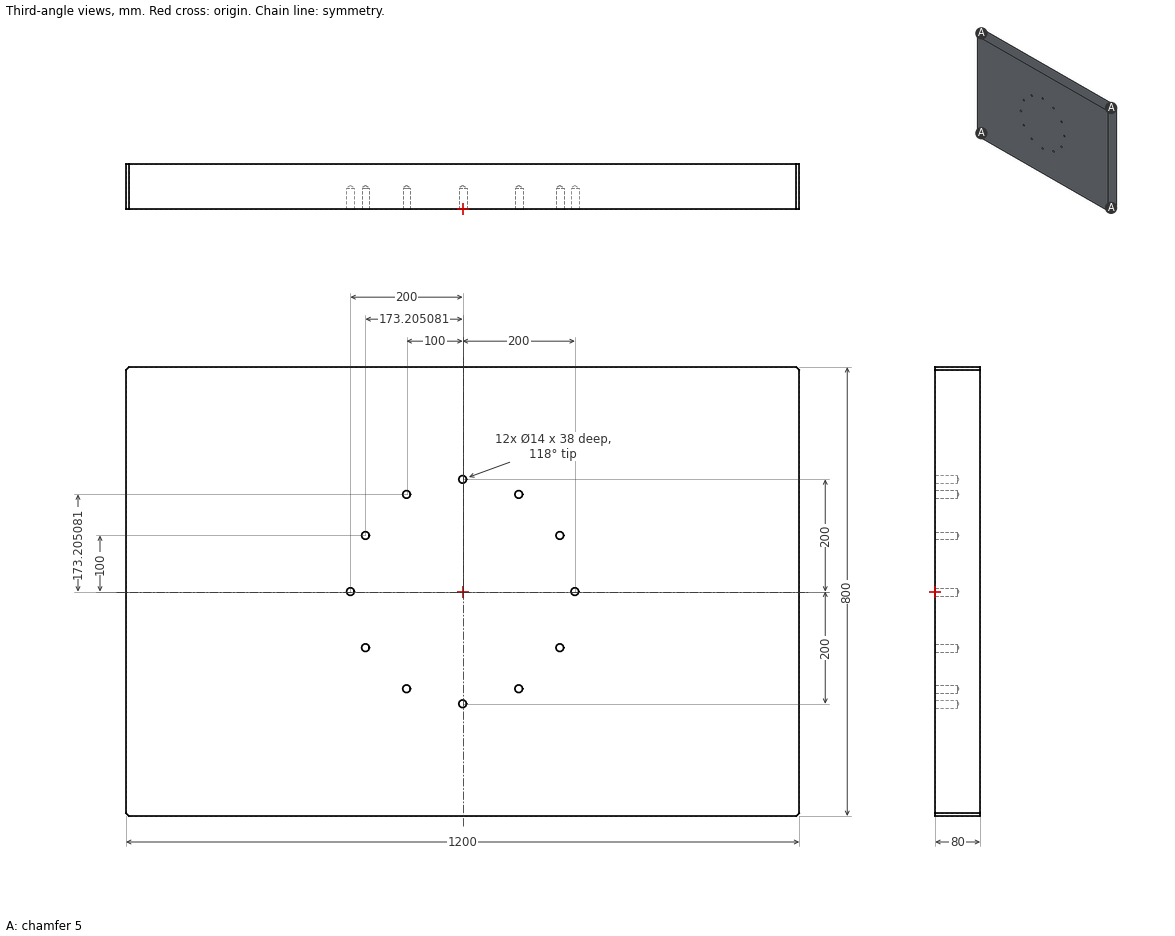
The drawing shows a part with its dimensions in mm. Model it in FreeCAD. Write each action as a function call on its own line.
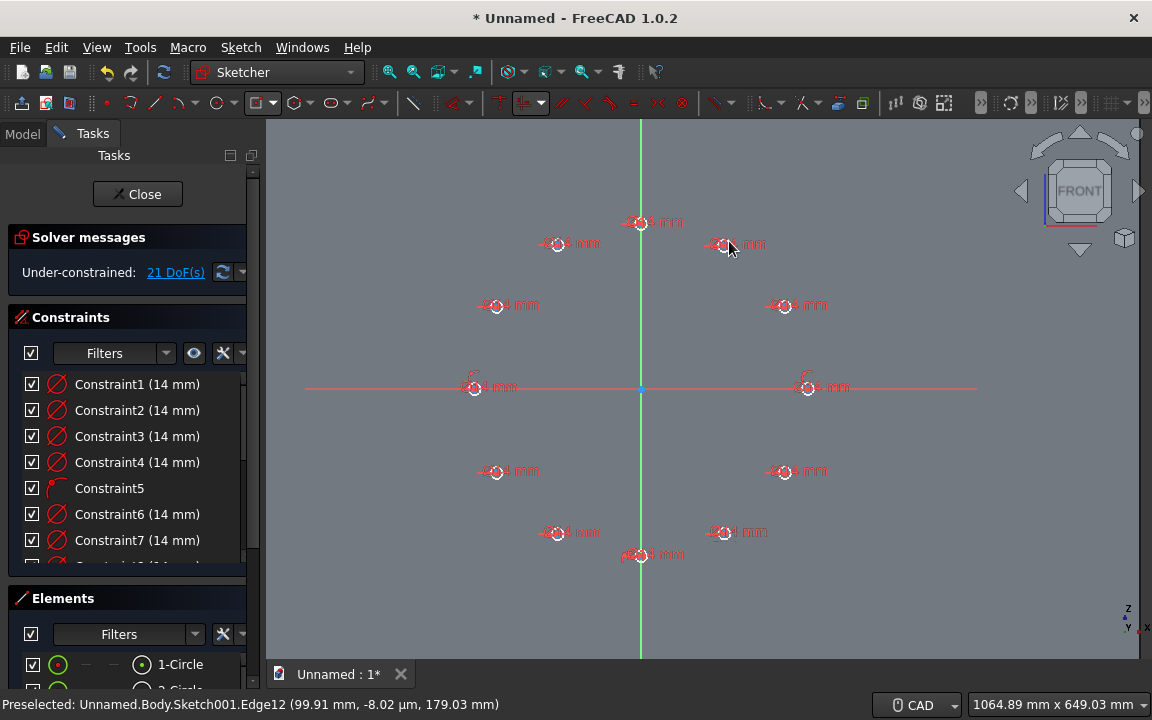
click(641, 224)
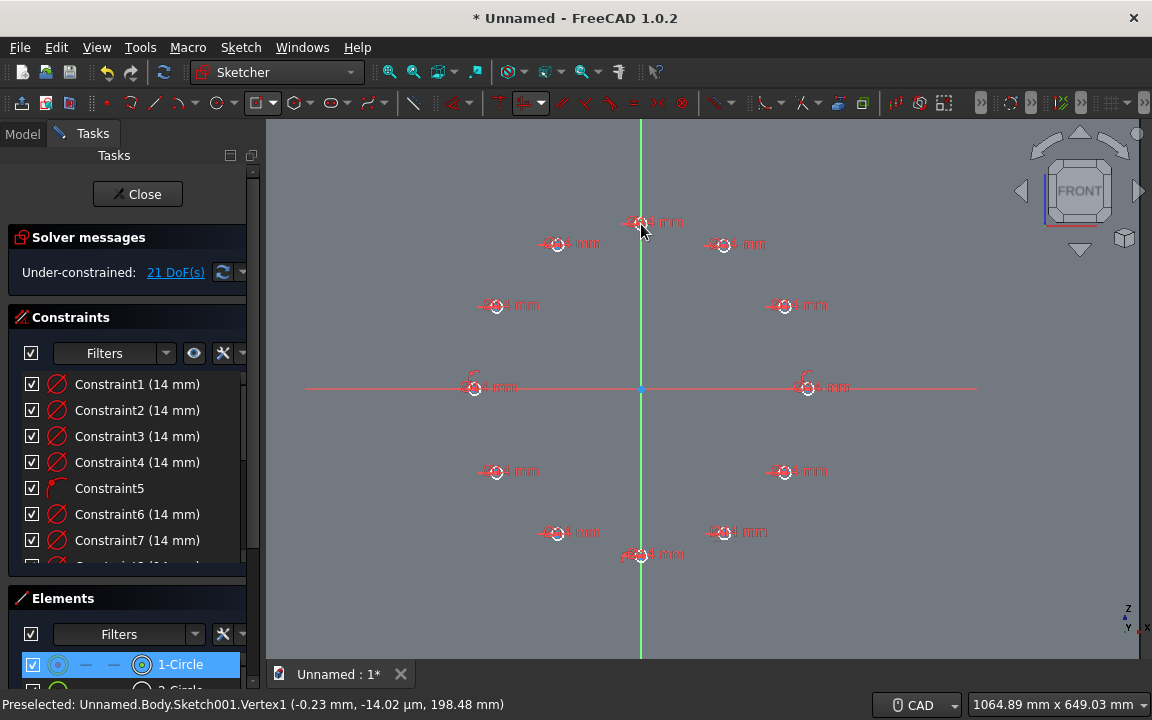
click(641, 596)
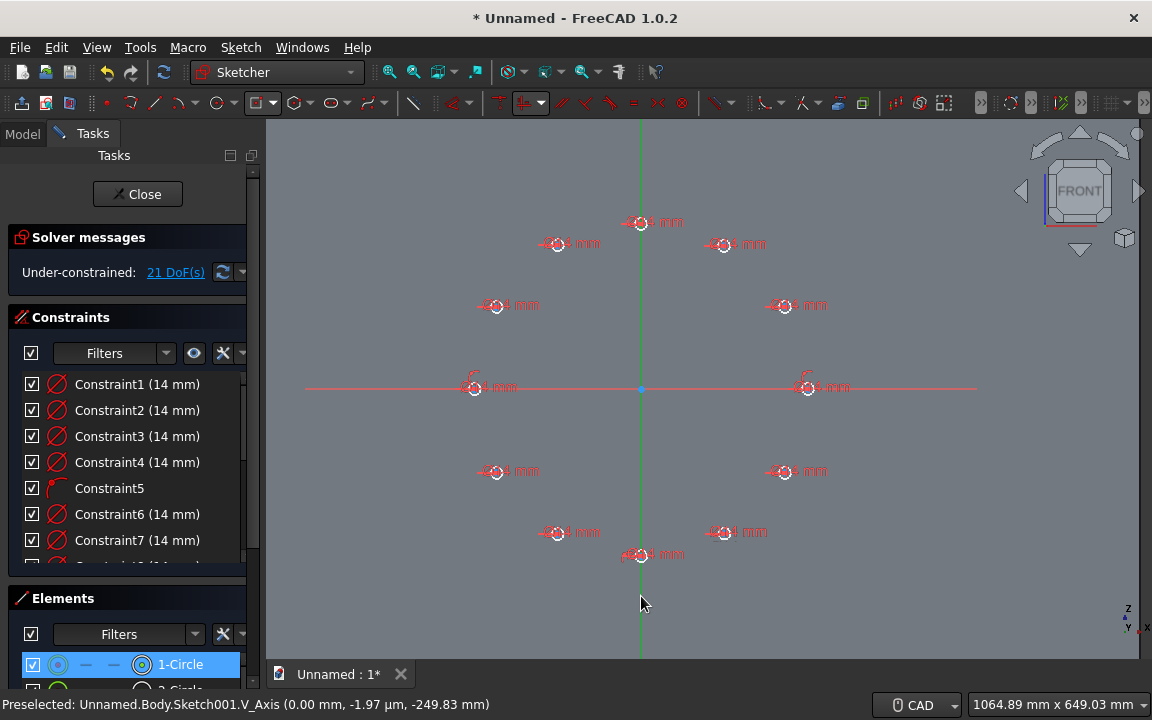
click(500, 104)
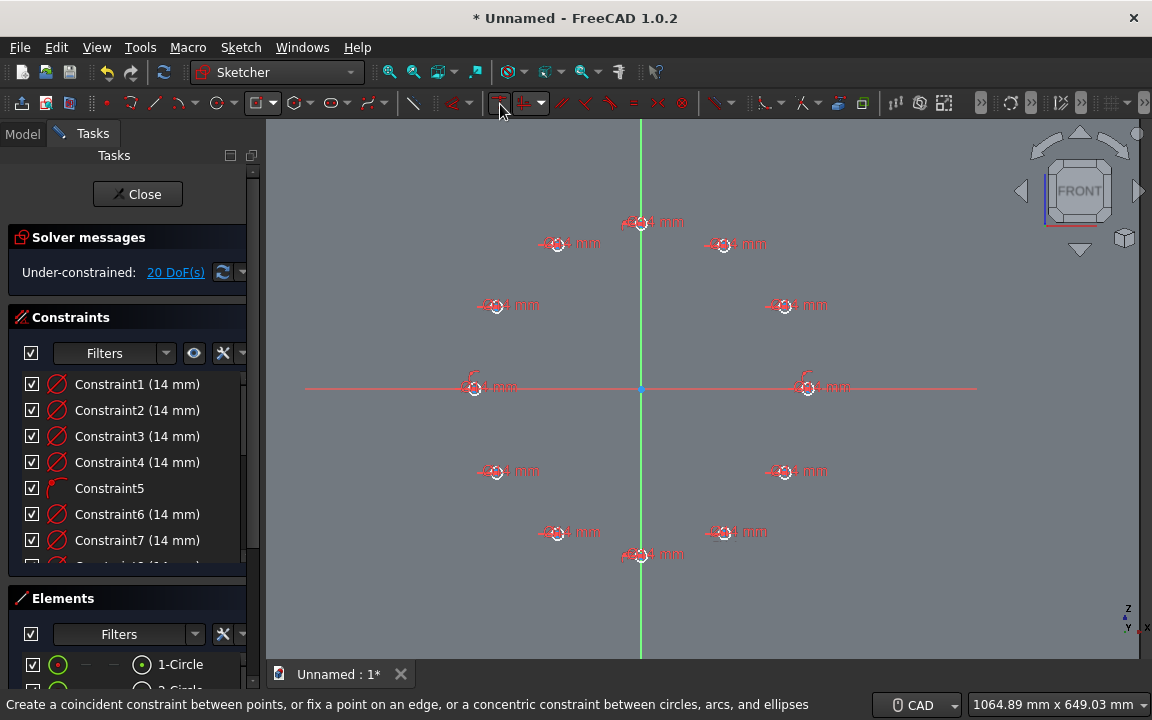
click(497, 307)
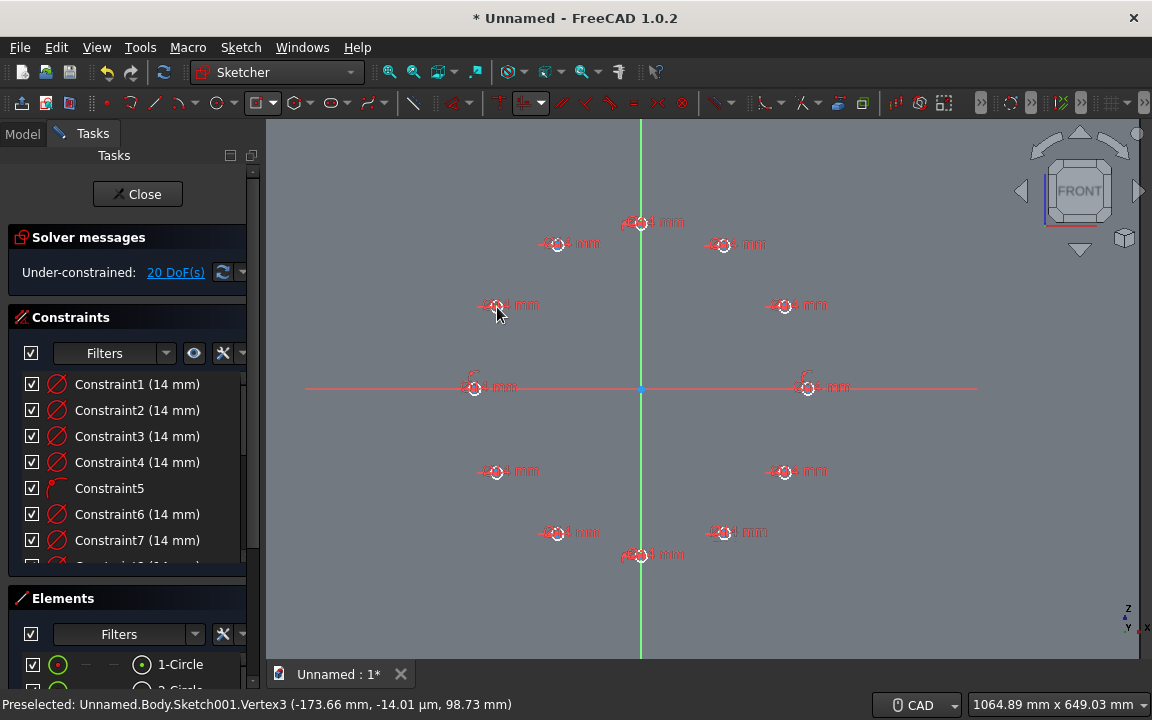
click(497, 473)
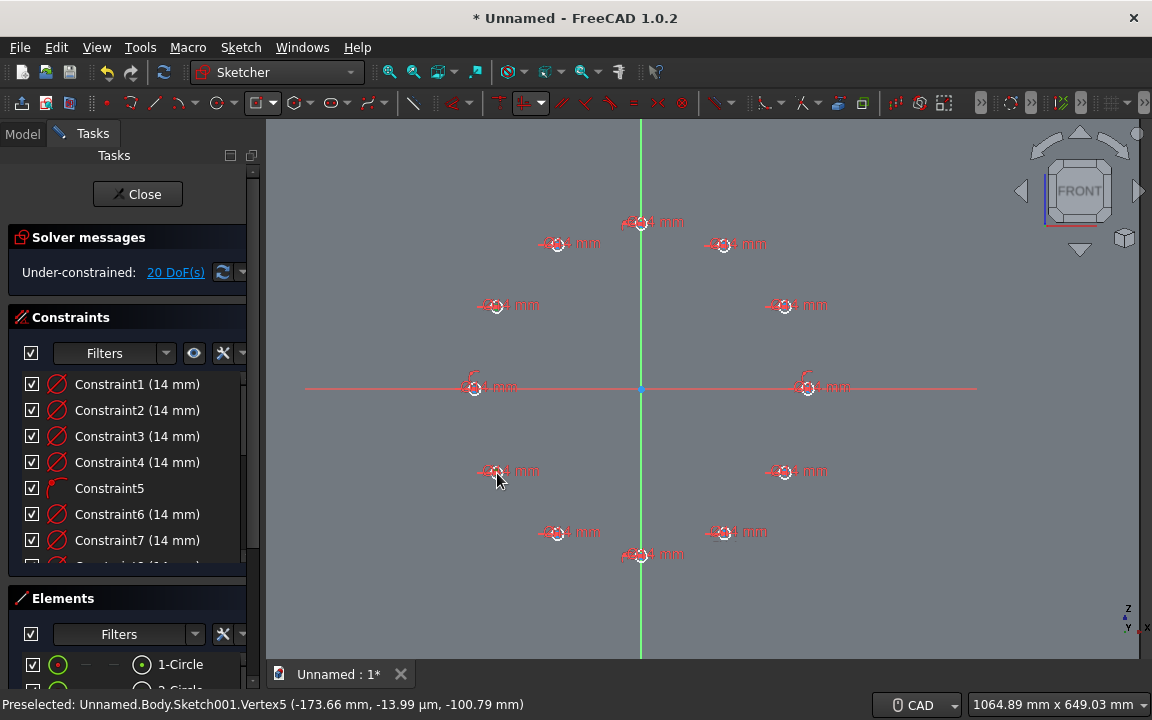
click(344, 389)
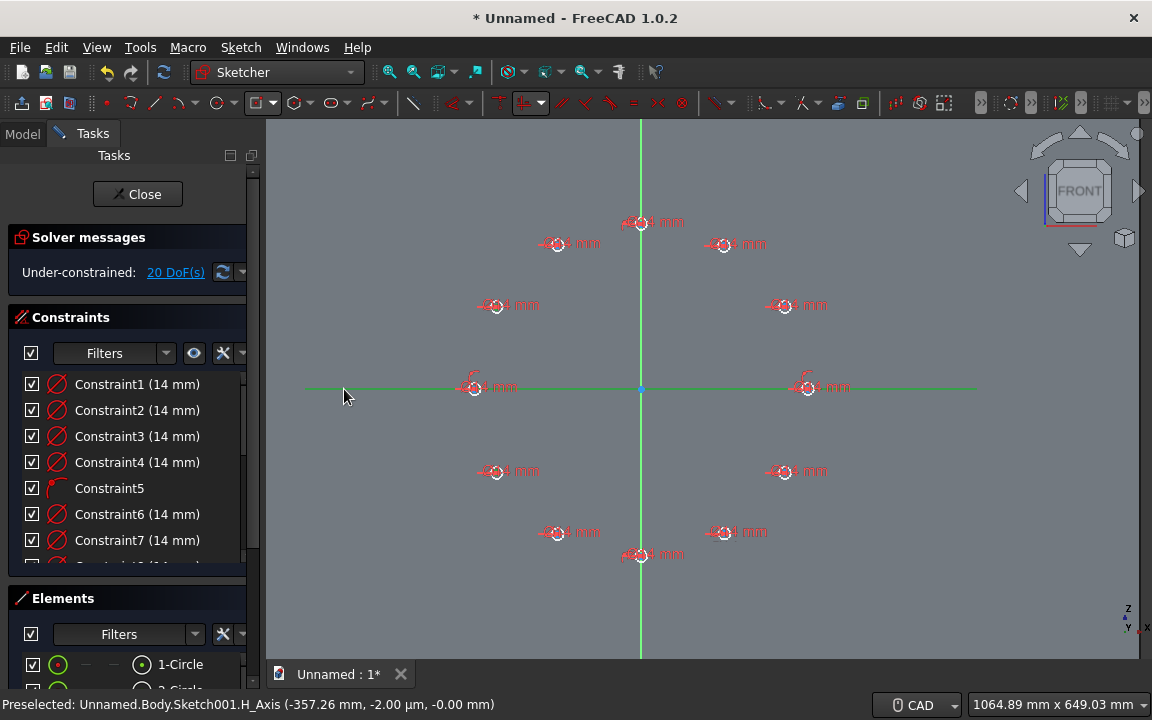
click(658, 104)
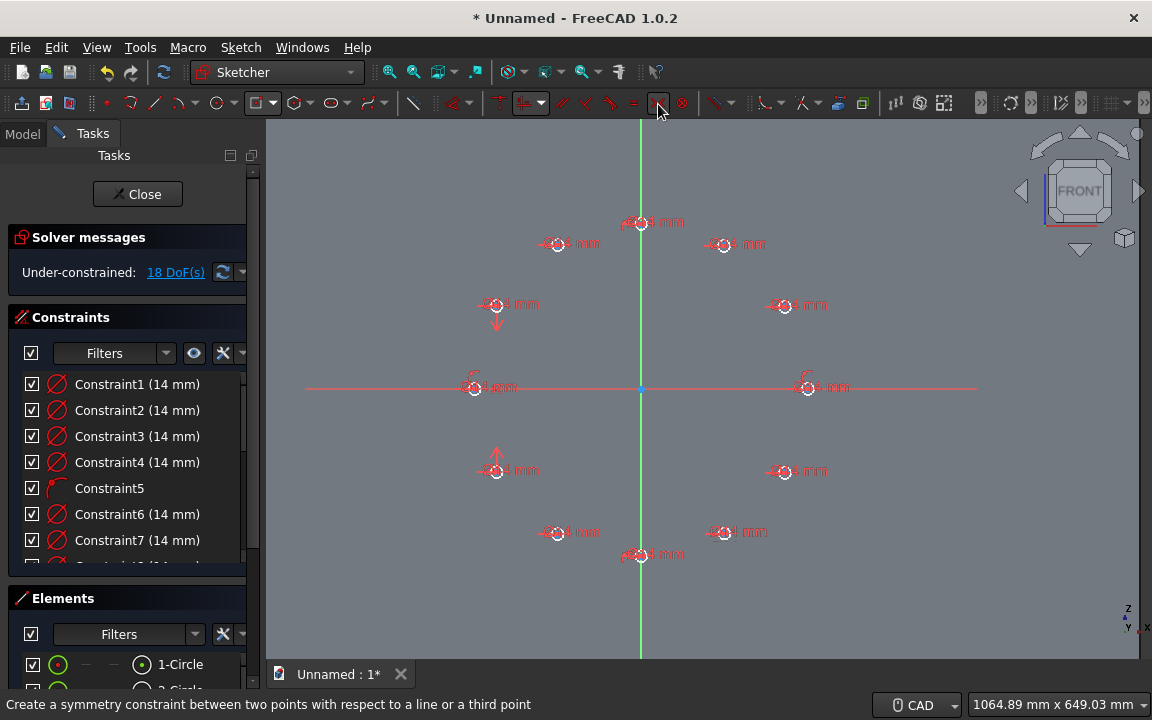
click(558, 245)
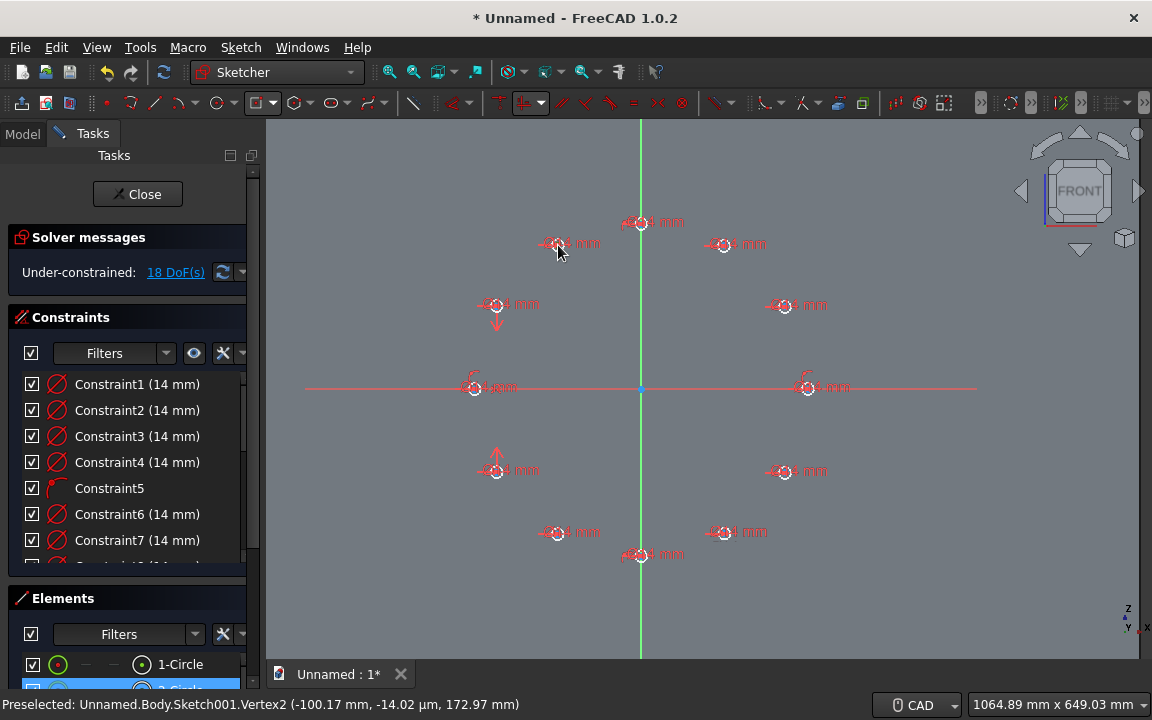
click(558, 534)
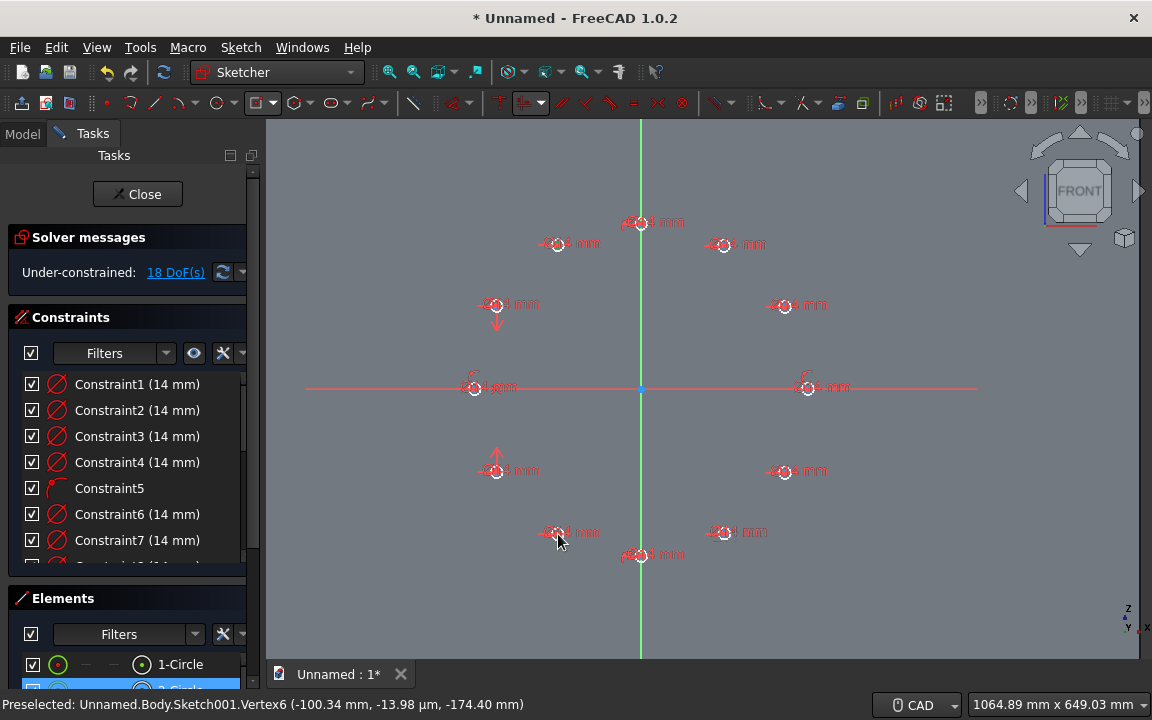
click(344, 389)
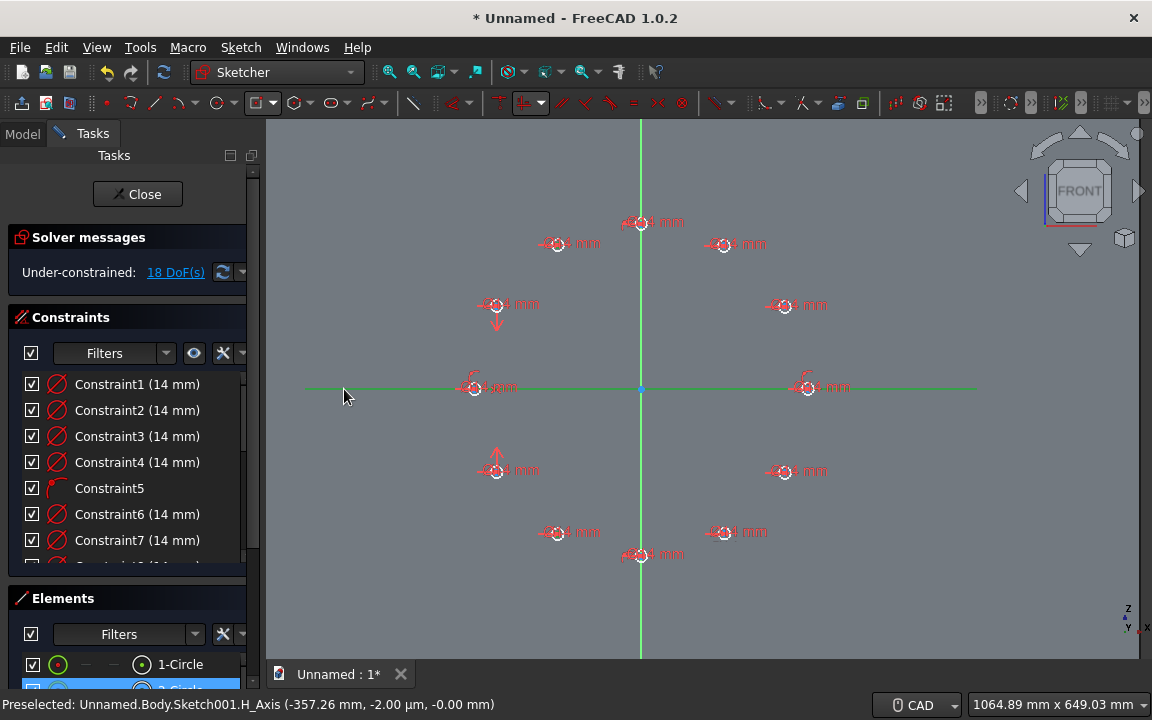
click(658, 104)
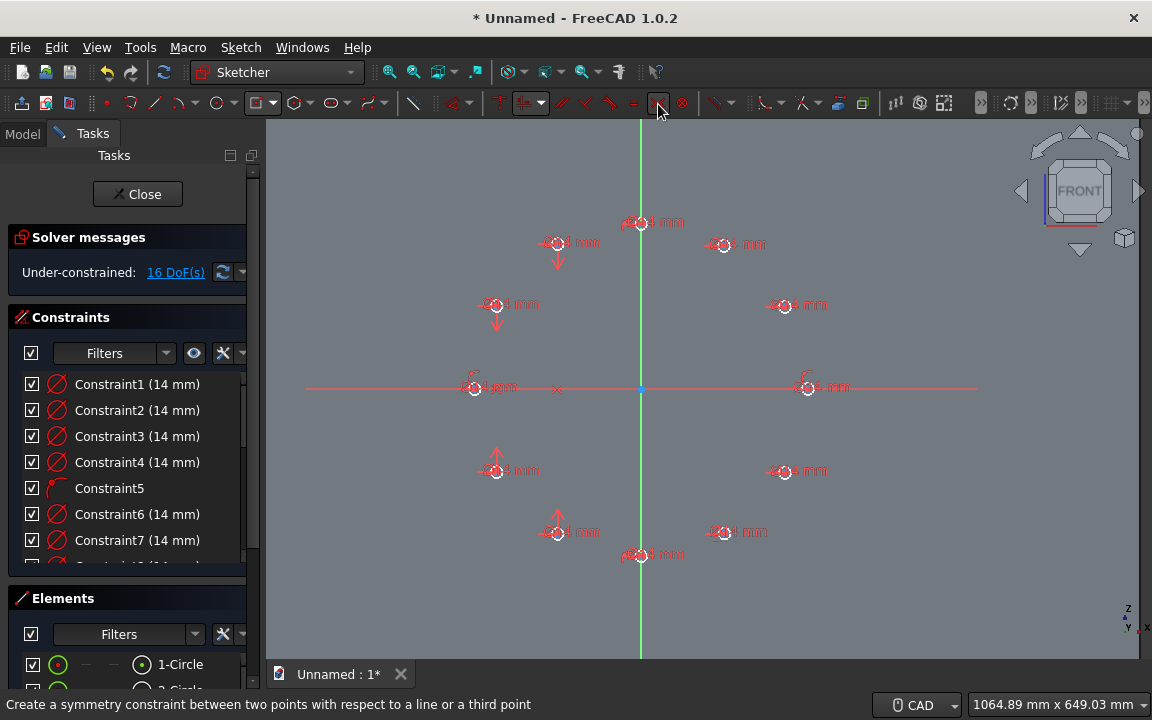
click(558, 534)